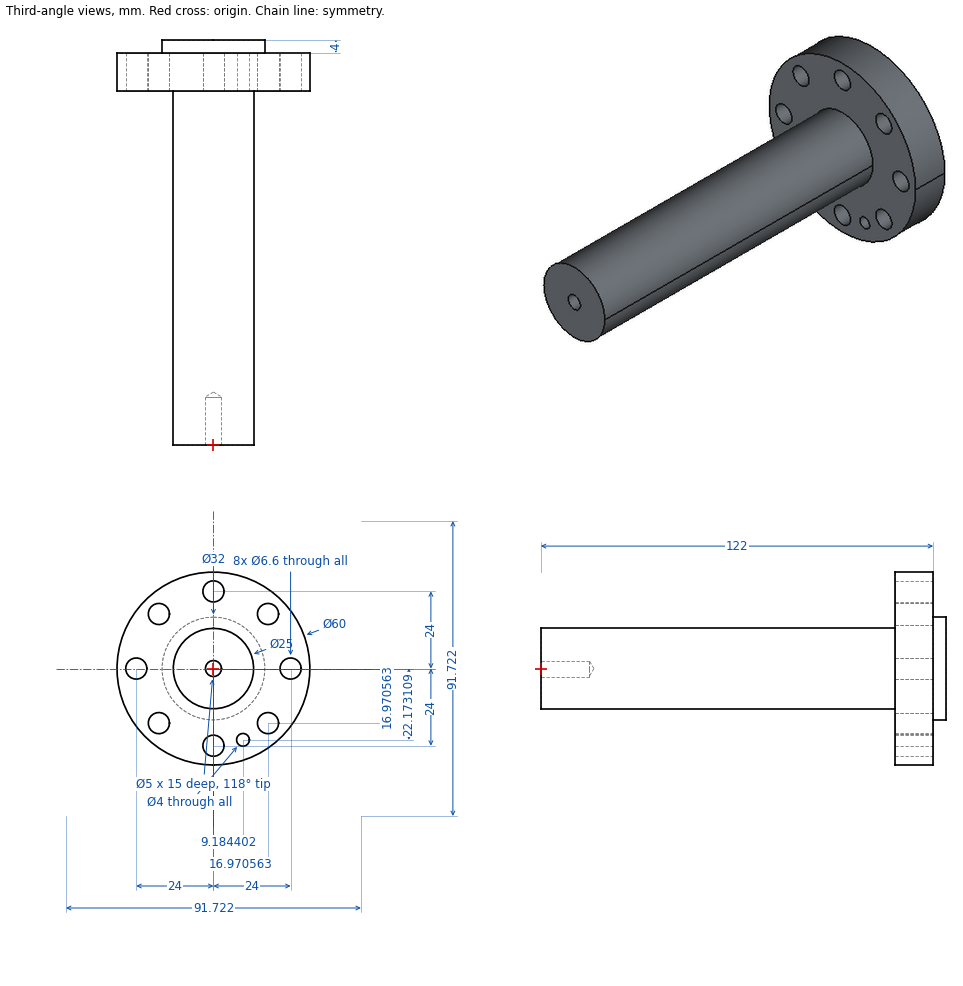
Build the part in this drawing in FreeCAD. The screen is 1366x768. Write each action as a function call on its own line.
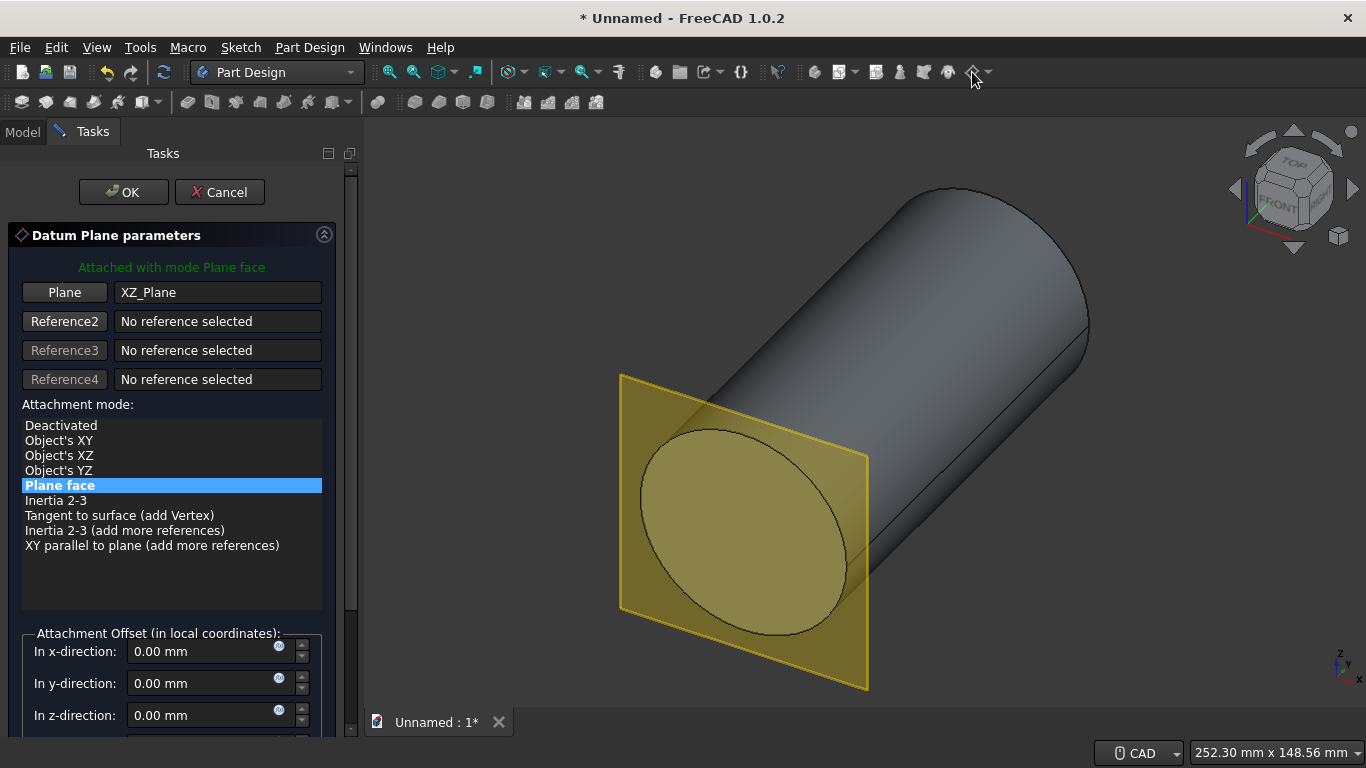
triple_click(210, 715)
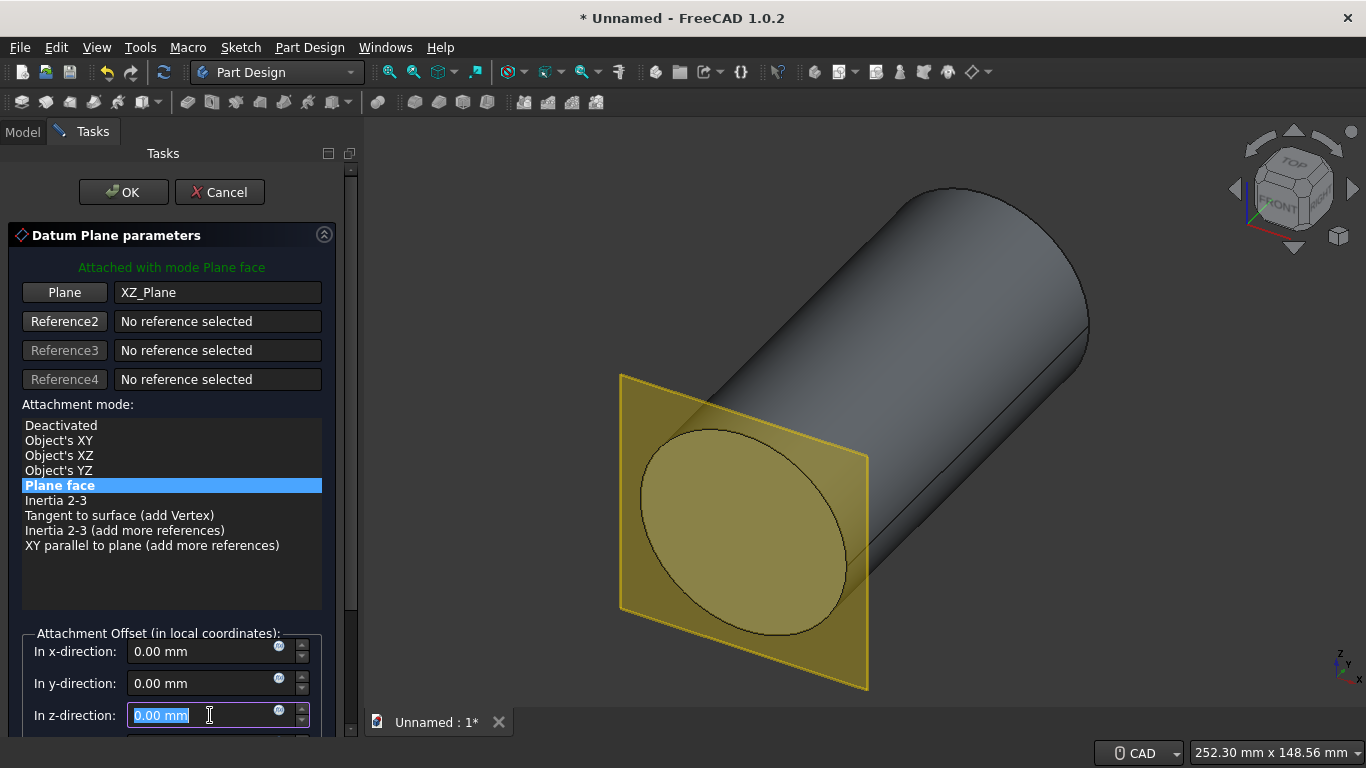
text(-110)
key(Tab)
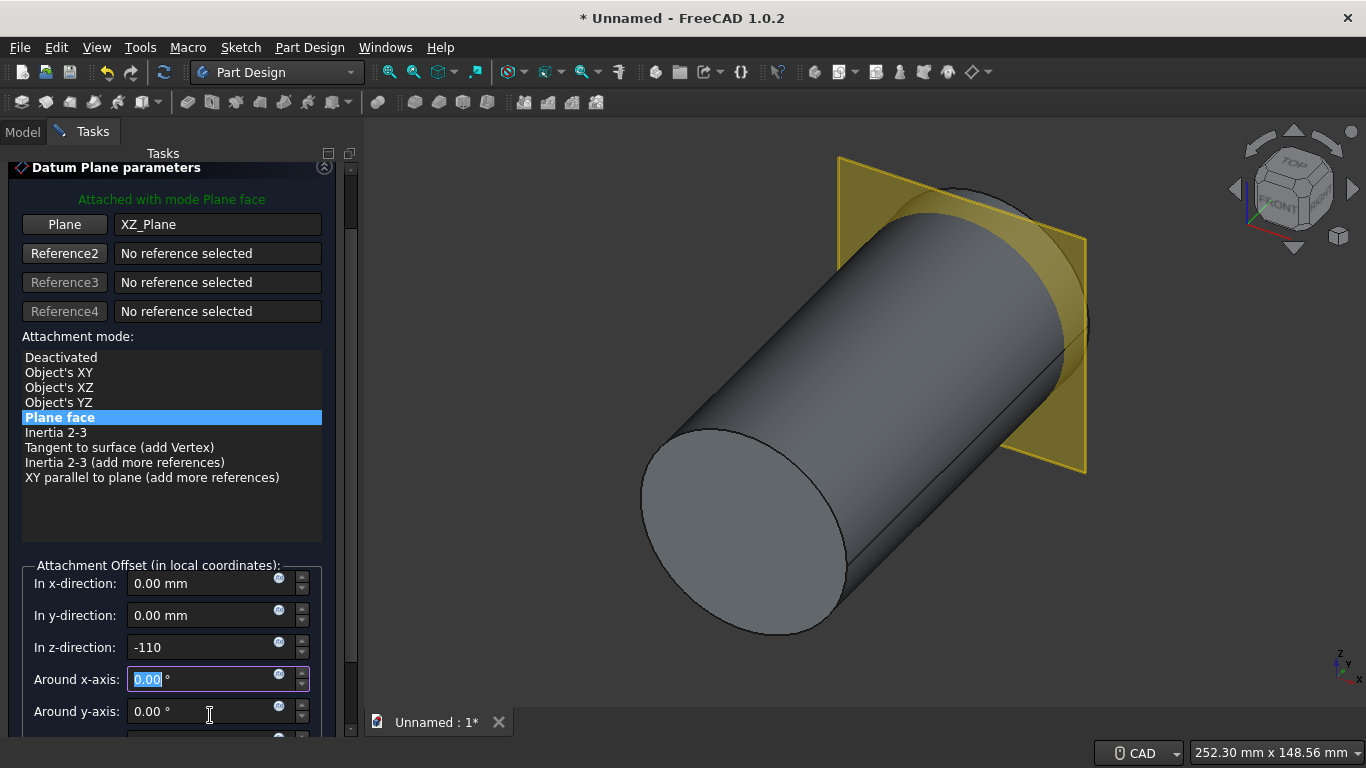
scroll(351, 450, up, 2)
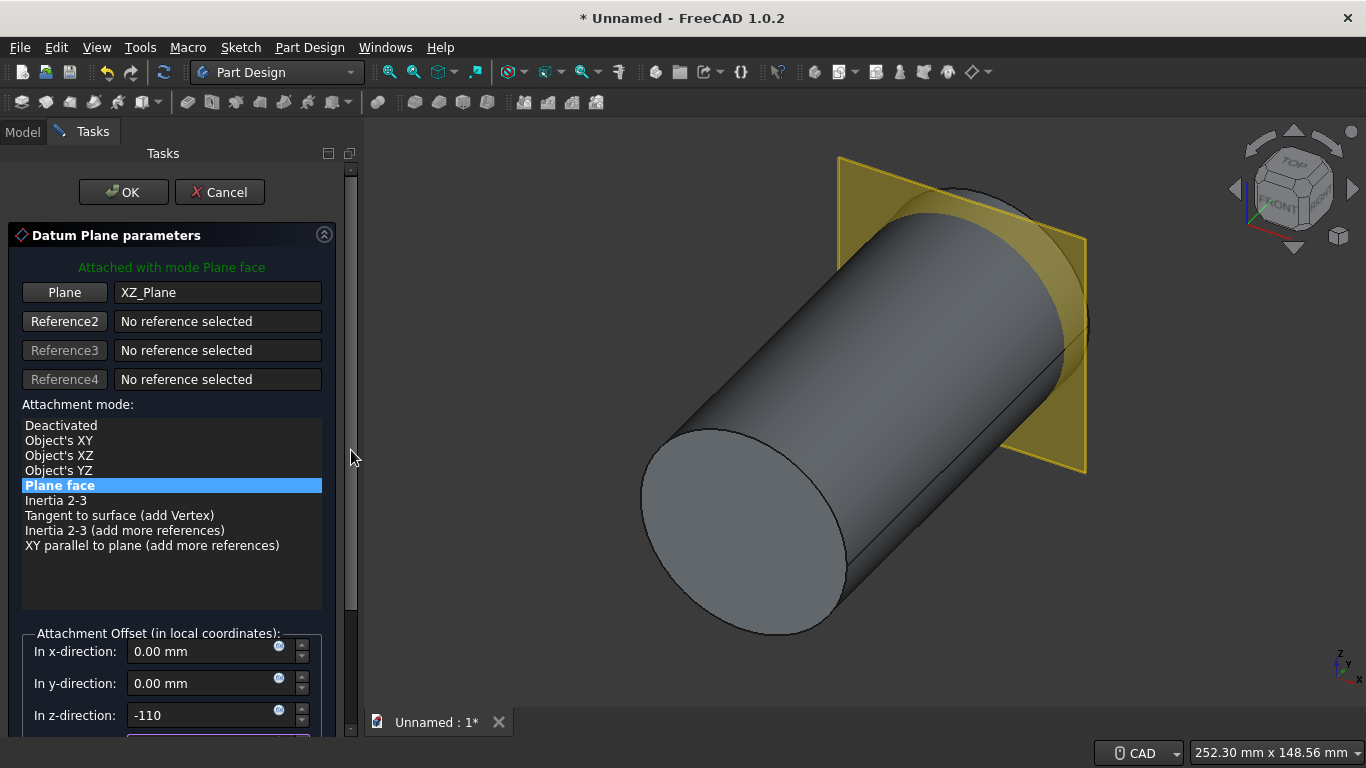
click(124, 192)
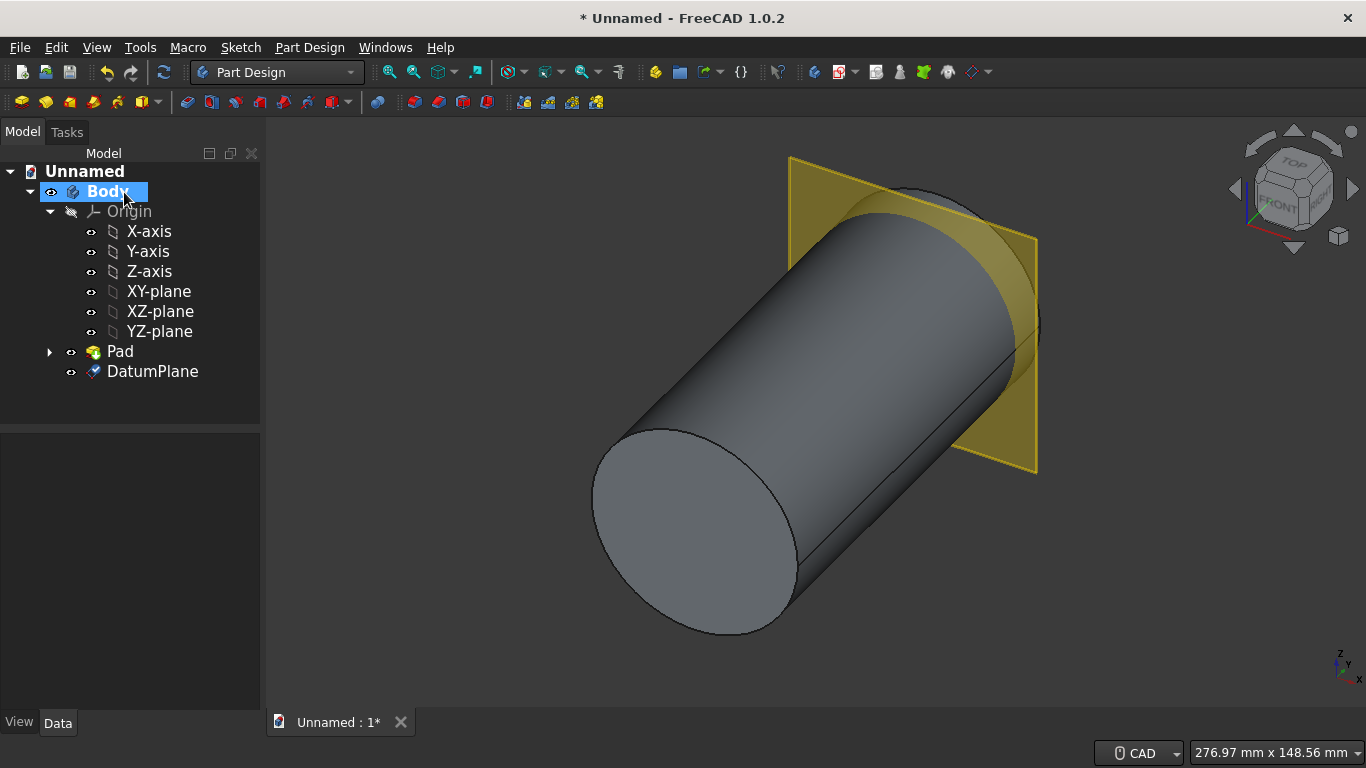
click(116, 372)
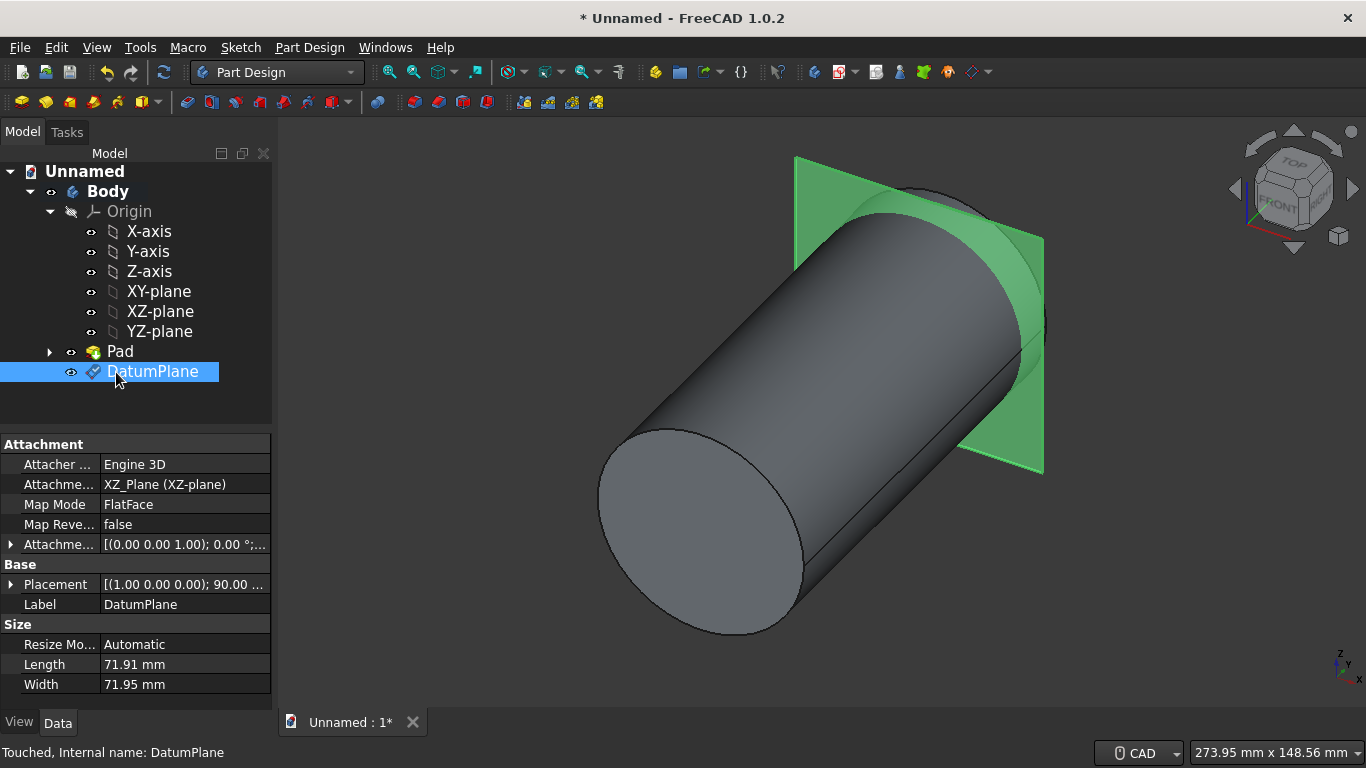
click(840, 72)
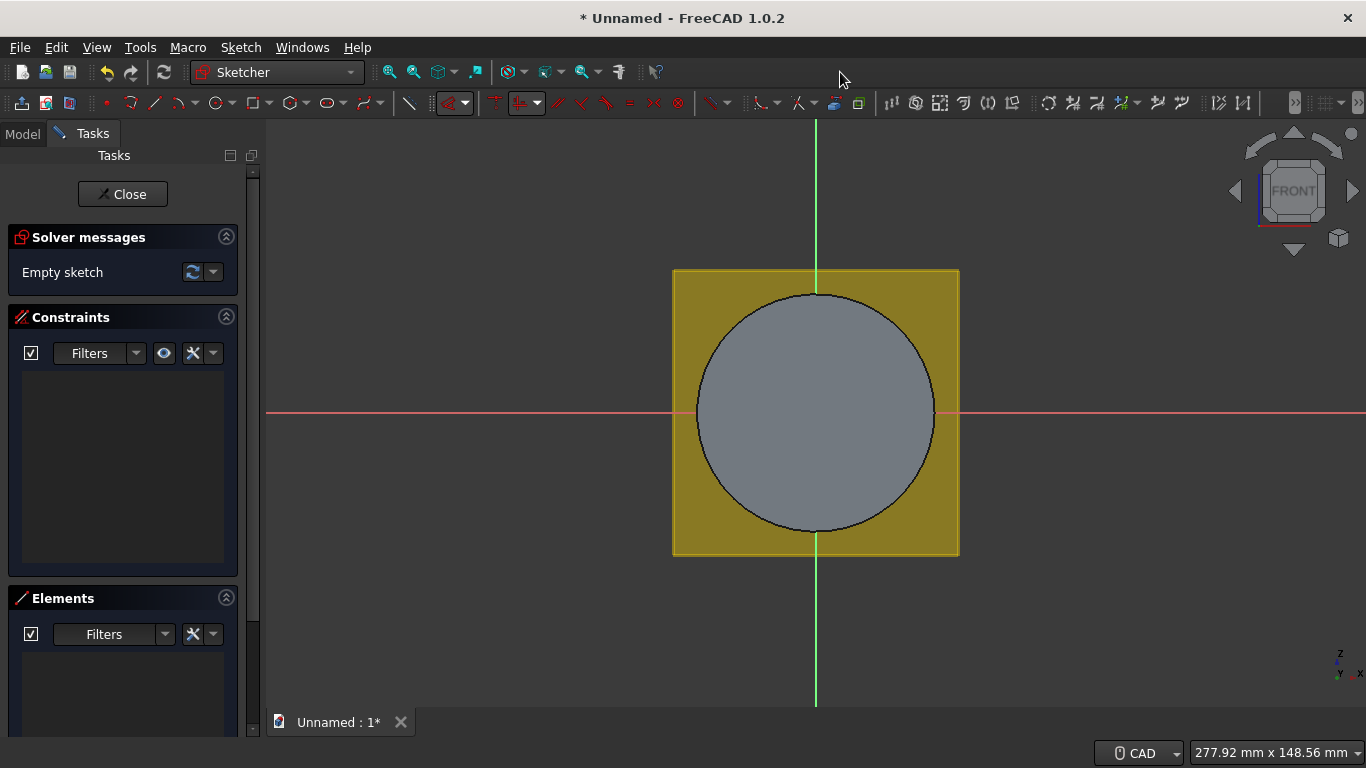
click(70, 104)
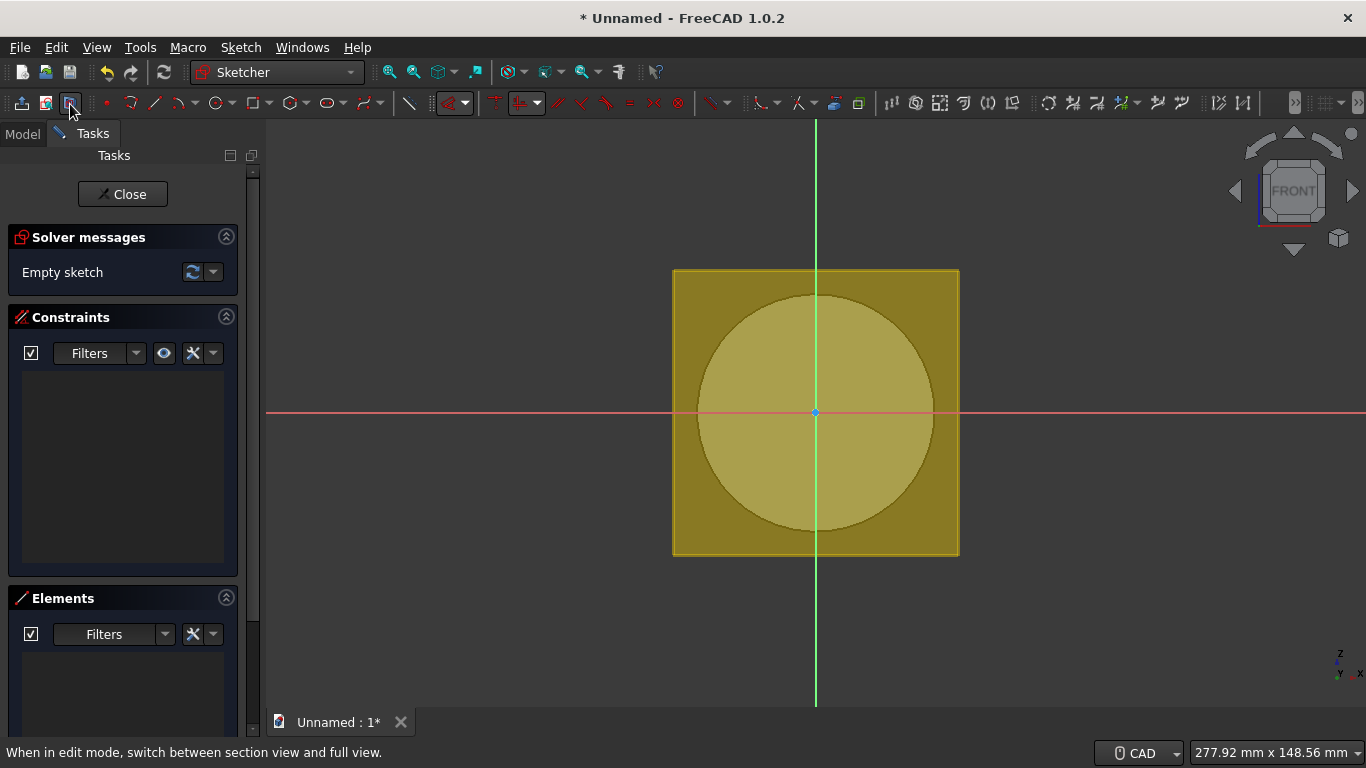
click(272, 104)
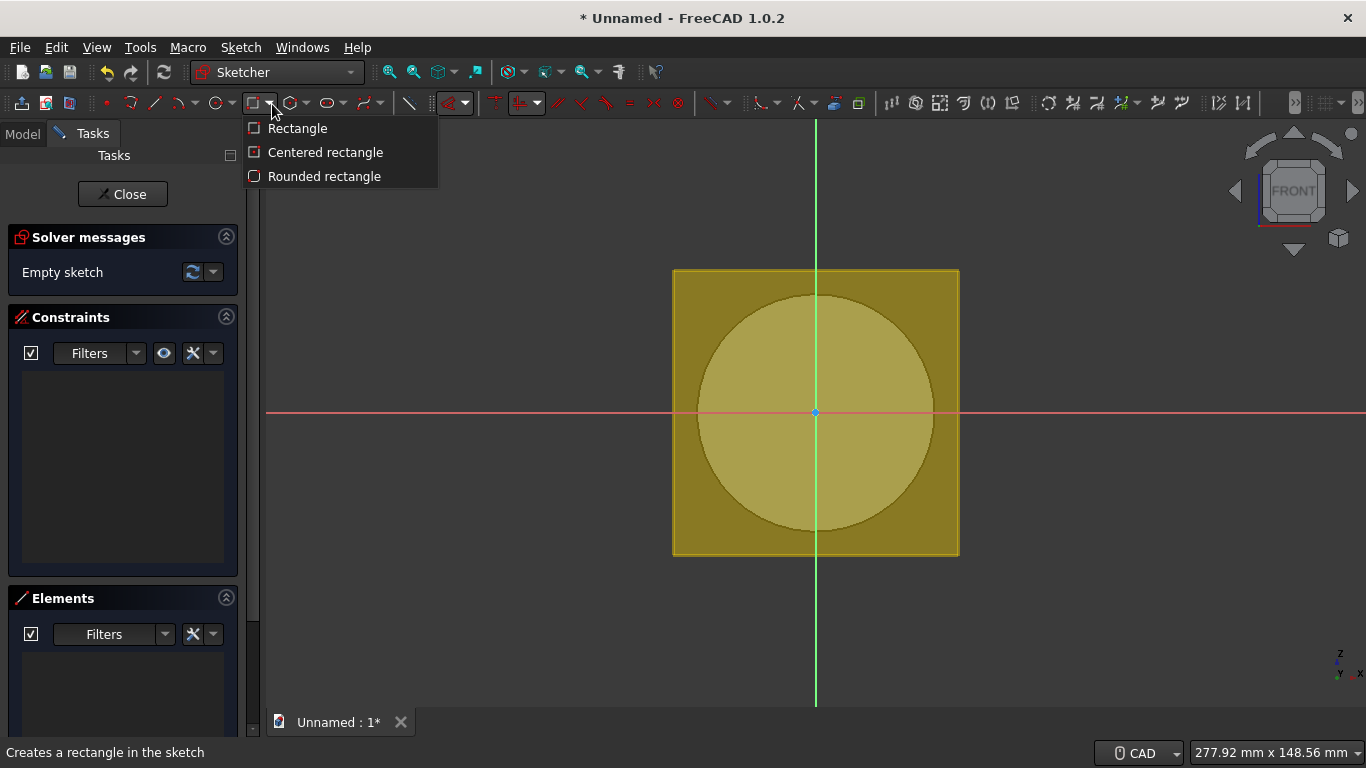
click(340, 152)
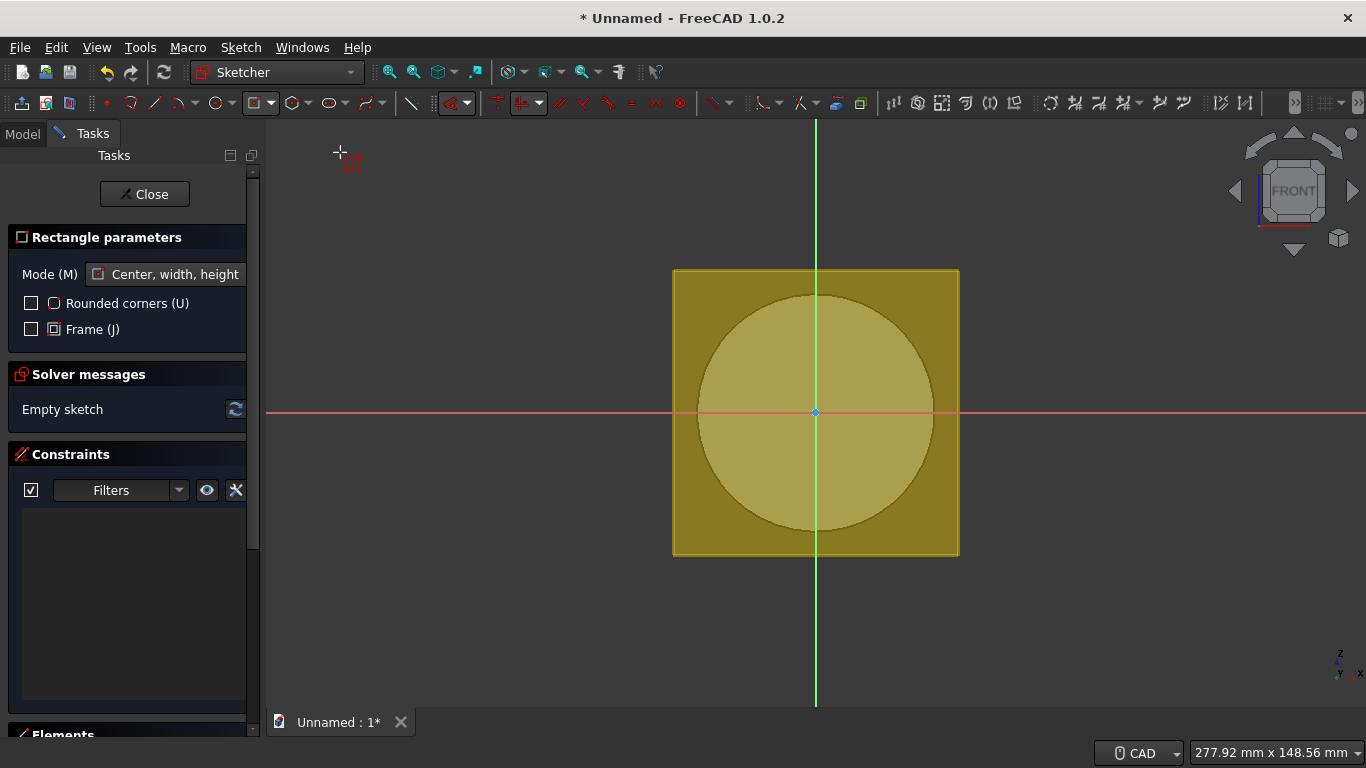
click(816, 413)
click(997, 231)